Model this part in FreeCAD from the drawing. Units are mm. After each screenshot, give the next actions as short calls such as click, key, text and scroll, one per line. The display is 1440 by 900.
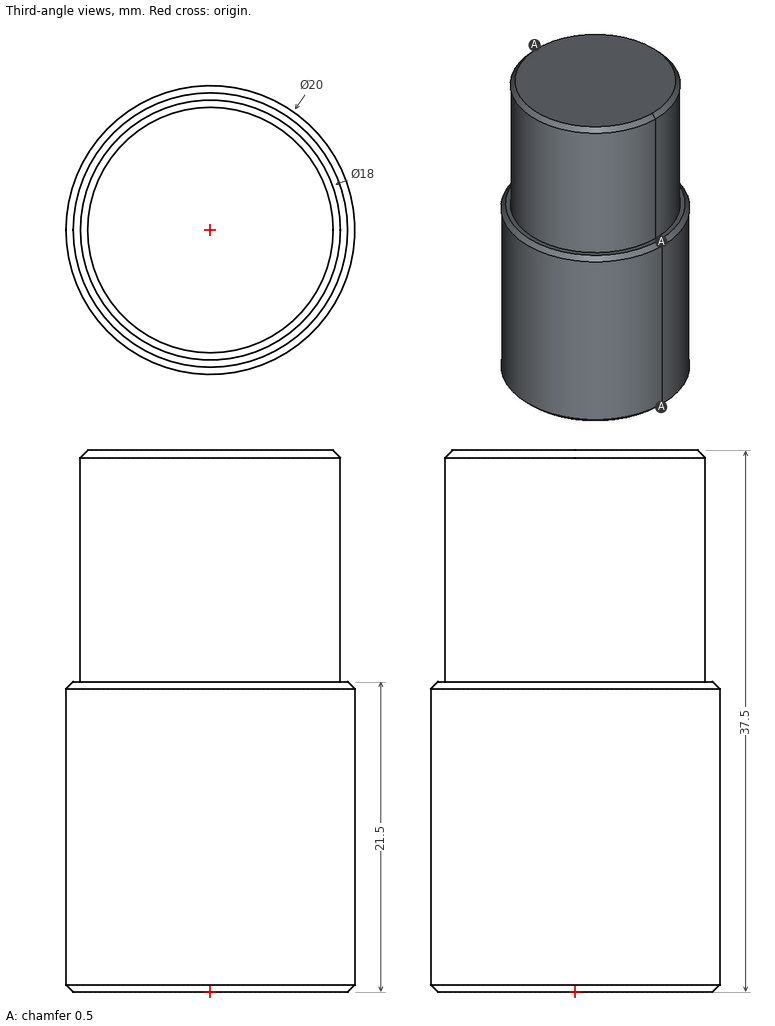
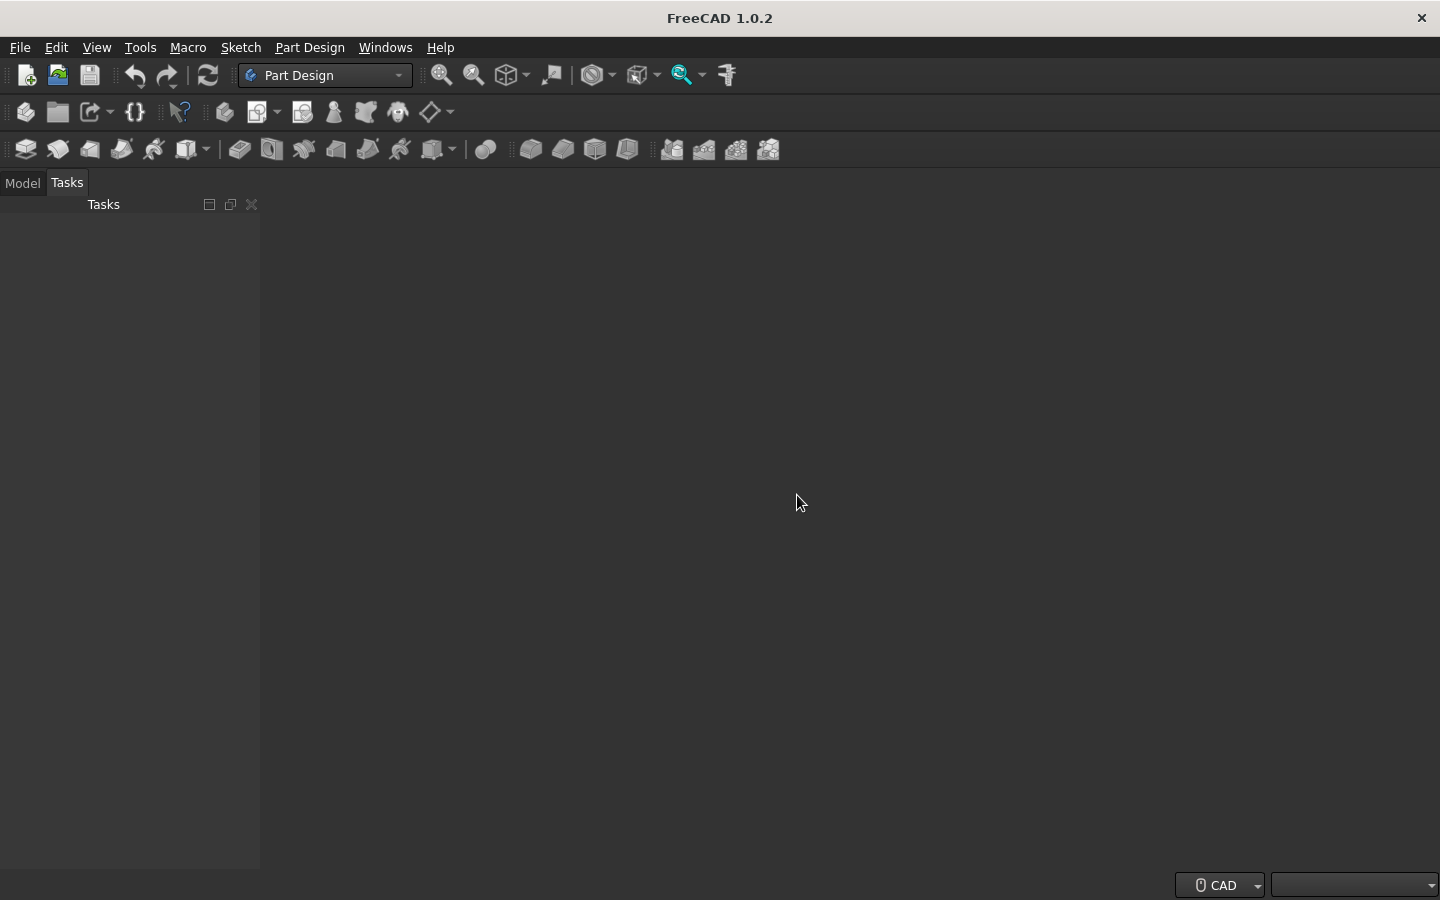
click(26, 76)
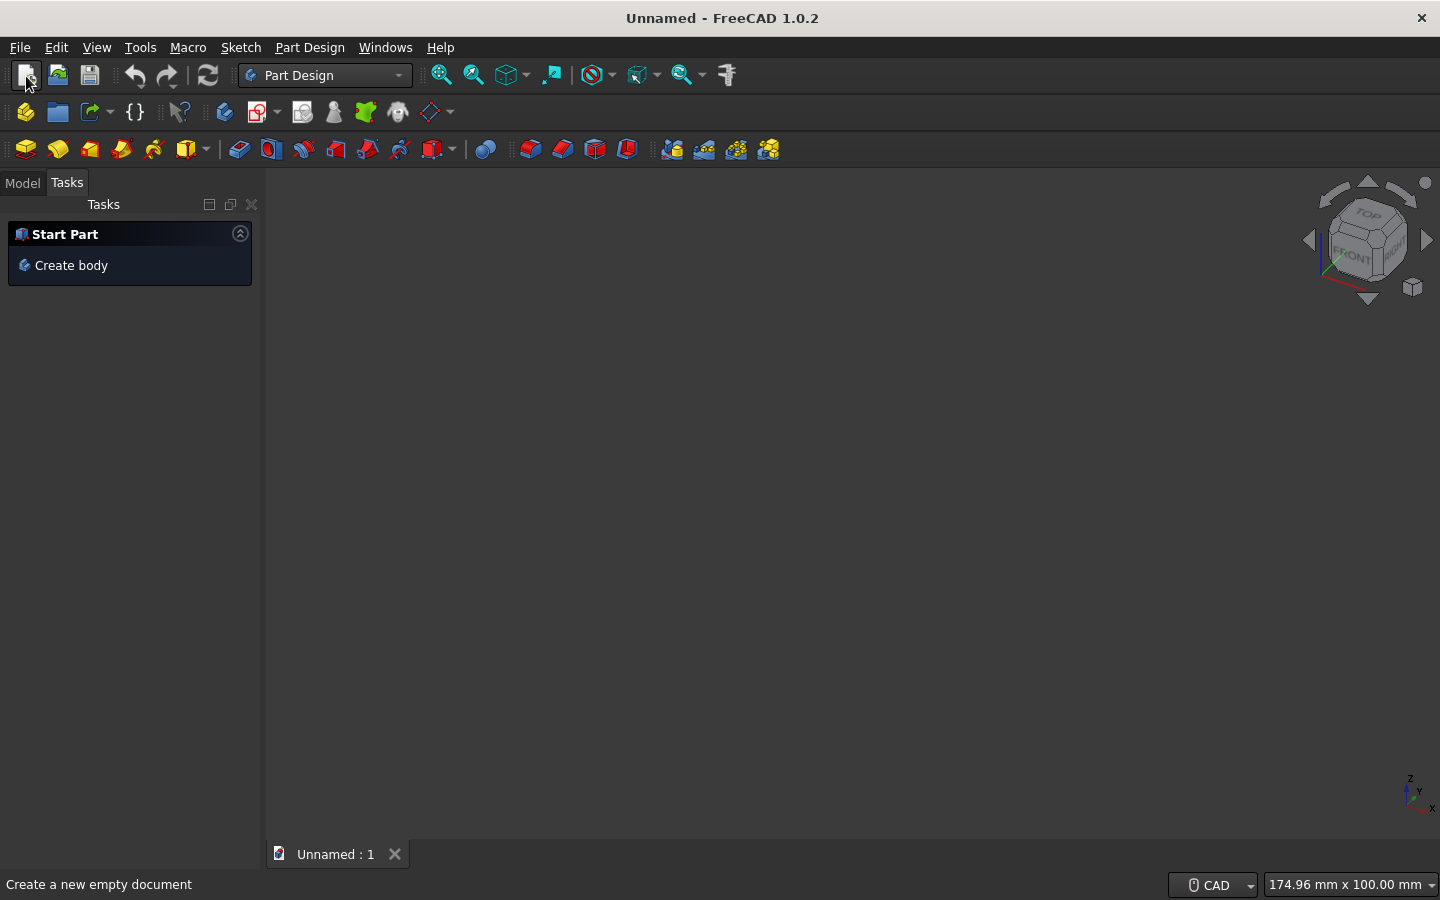
click(258, 112)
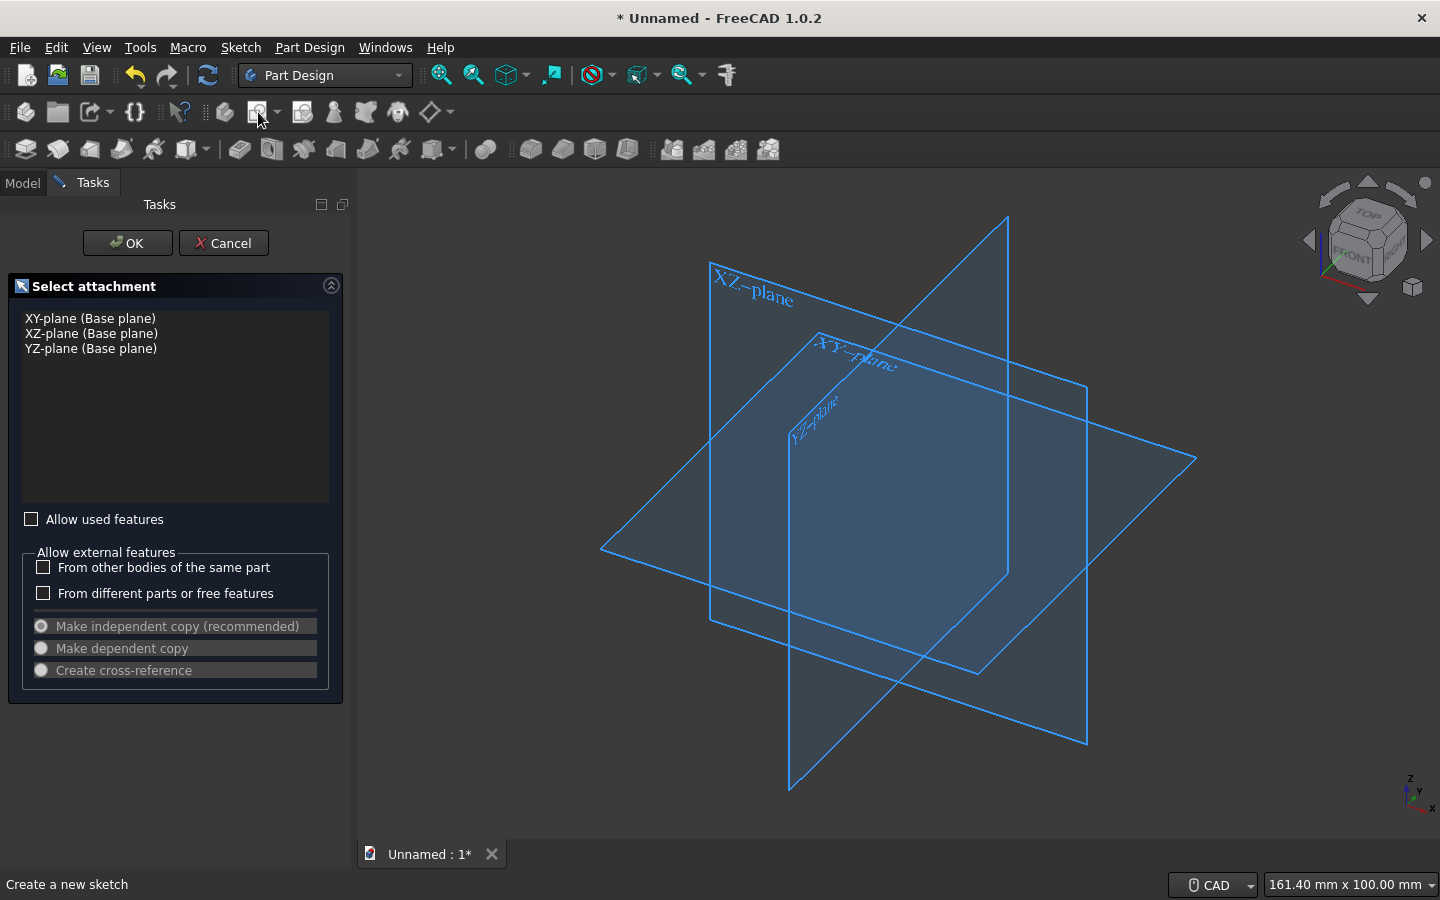
click(82, 318)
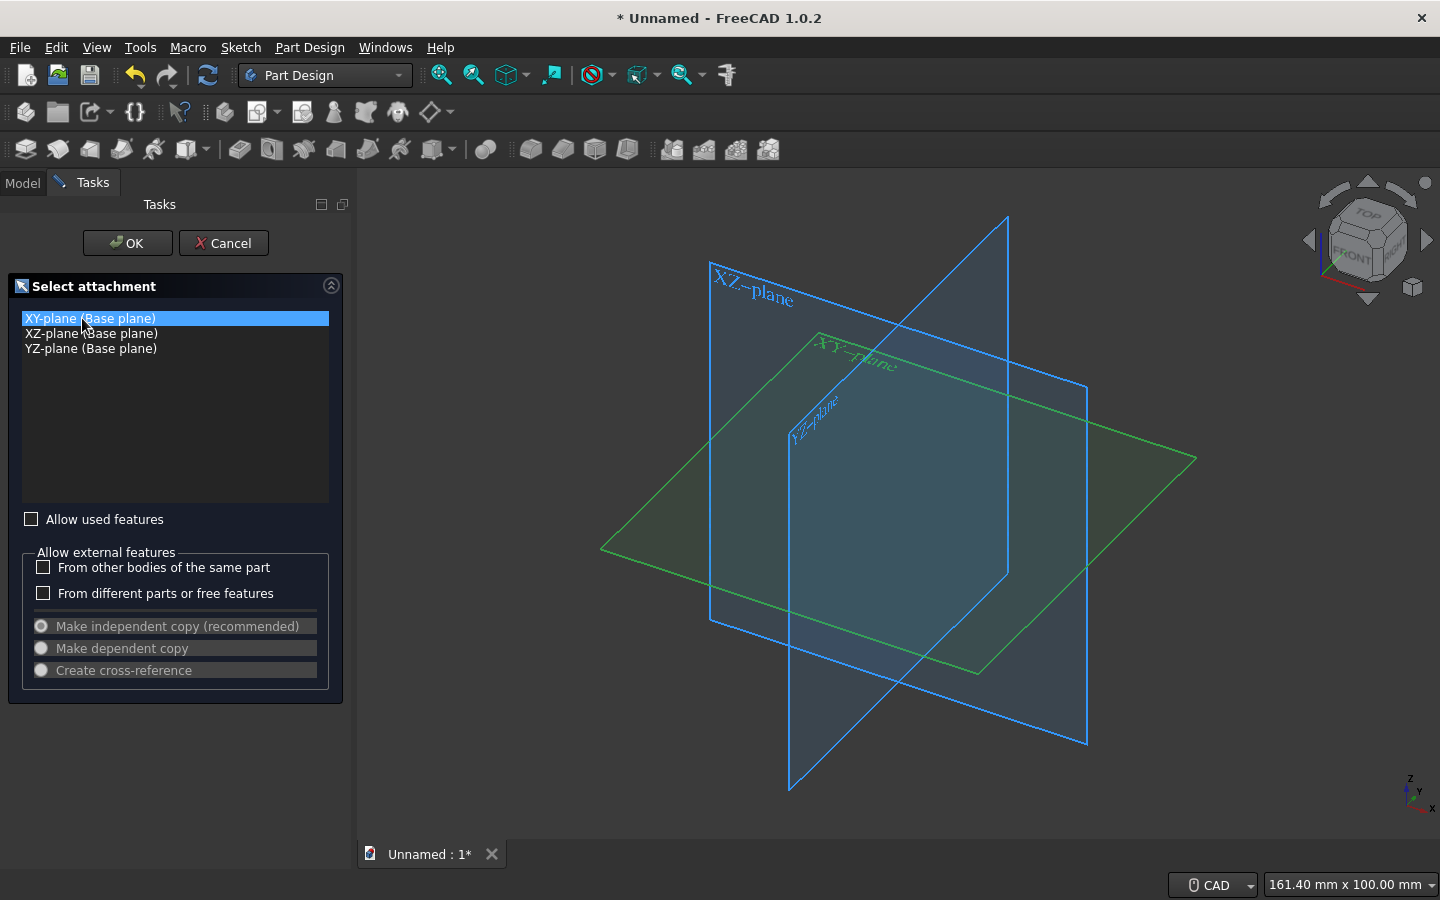
click(128, 243)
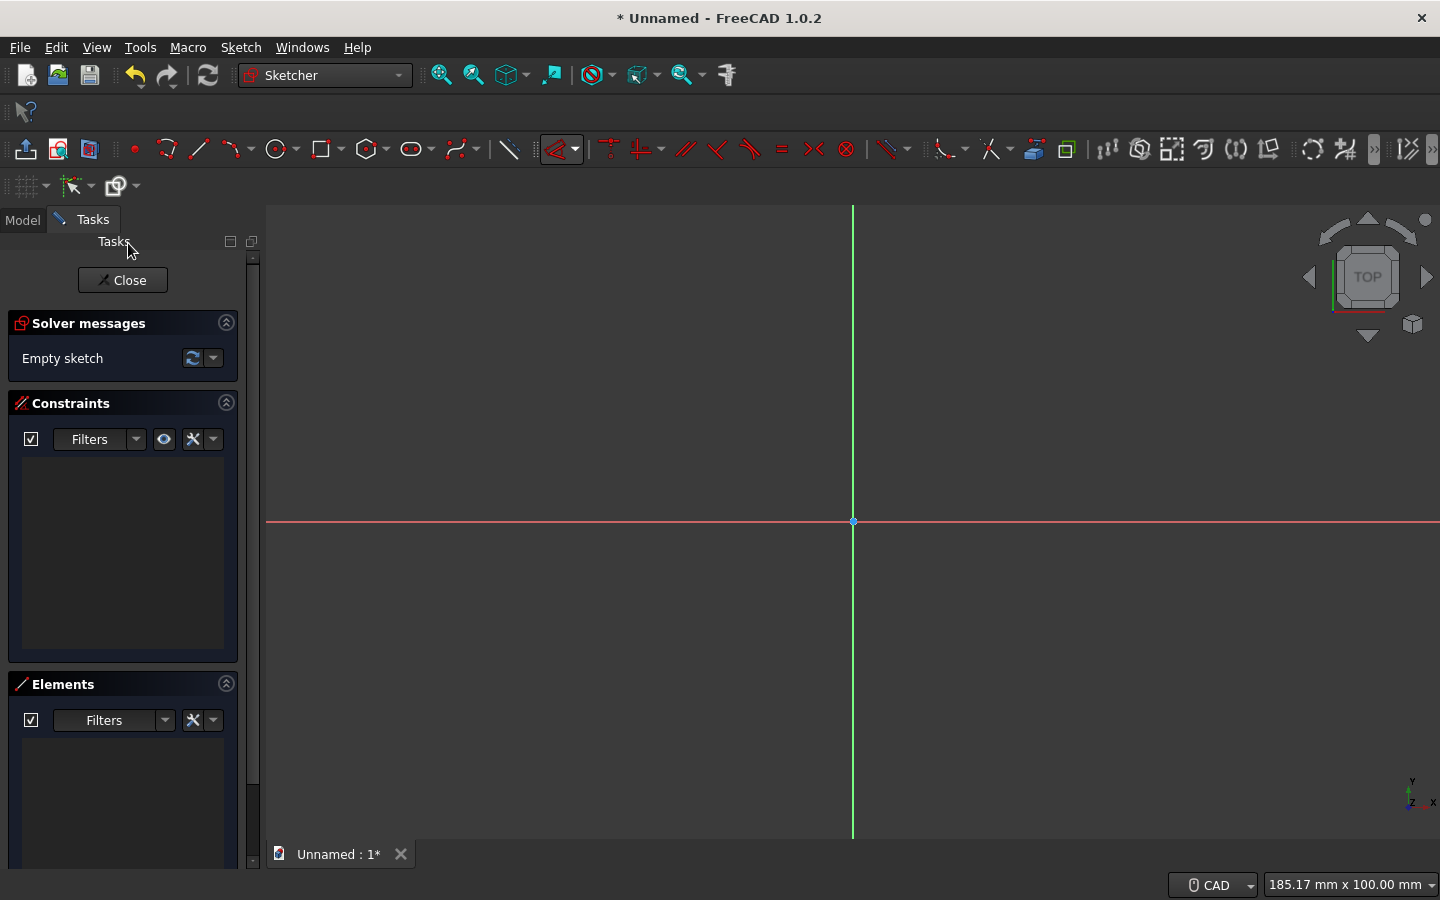
scroll(883, 522, up, 6)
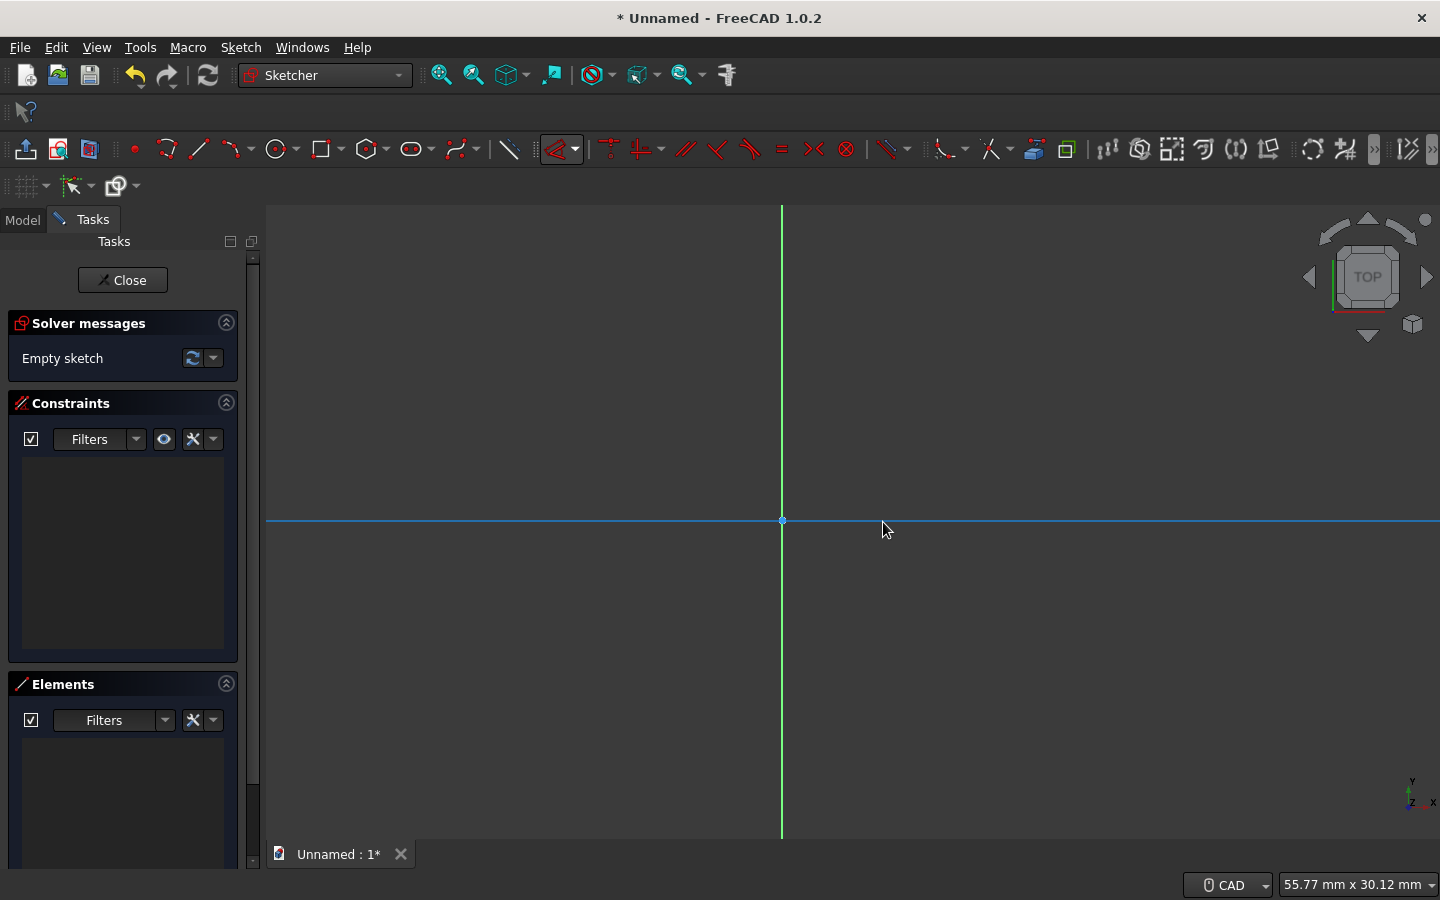
click(276, 150)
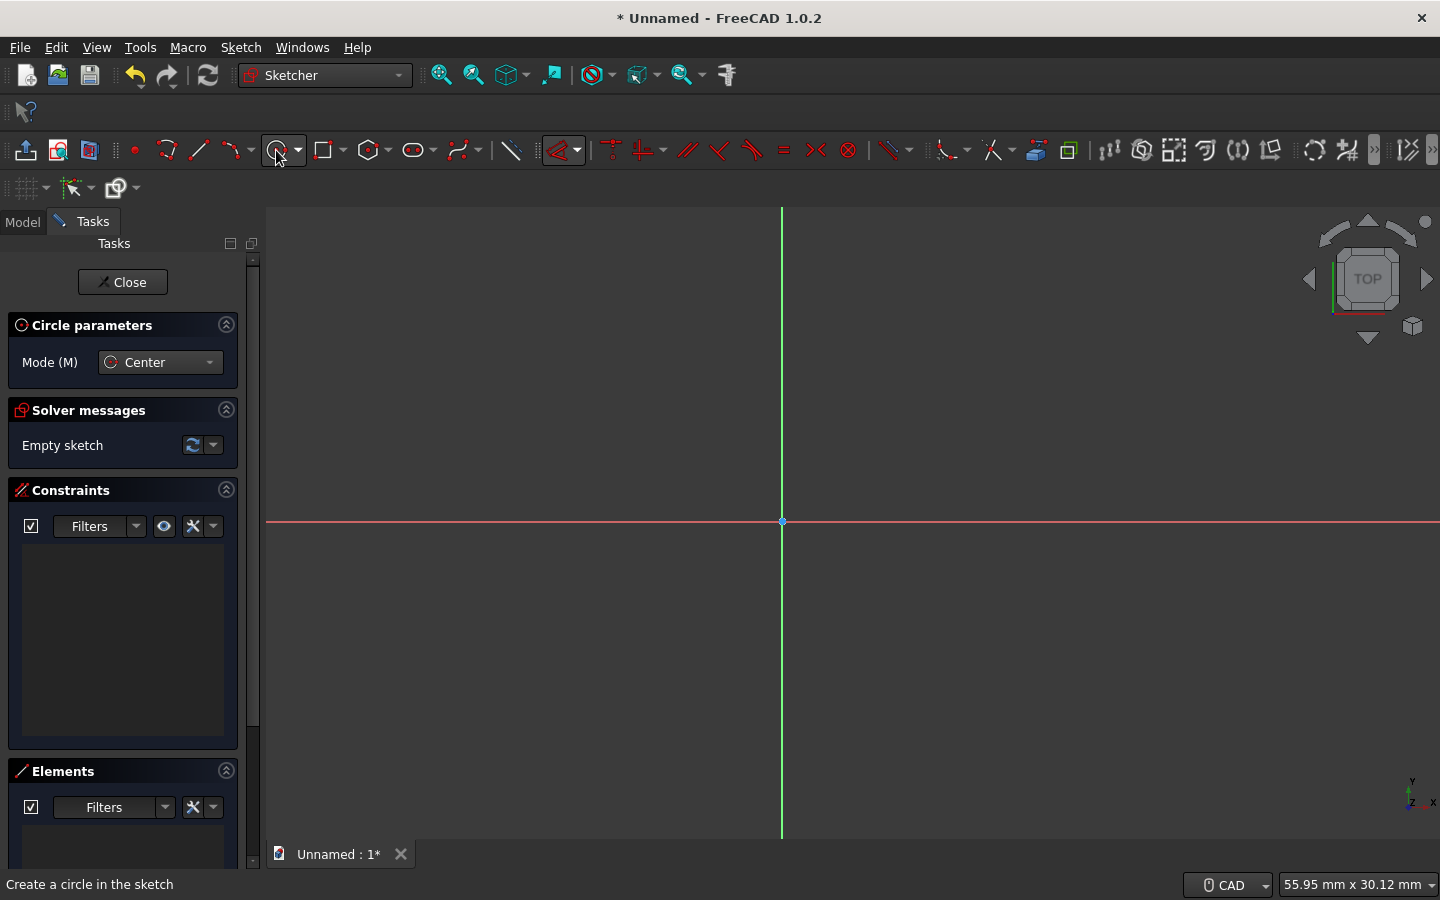
click(782, 522)
move(916, 388)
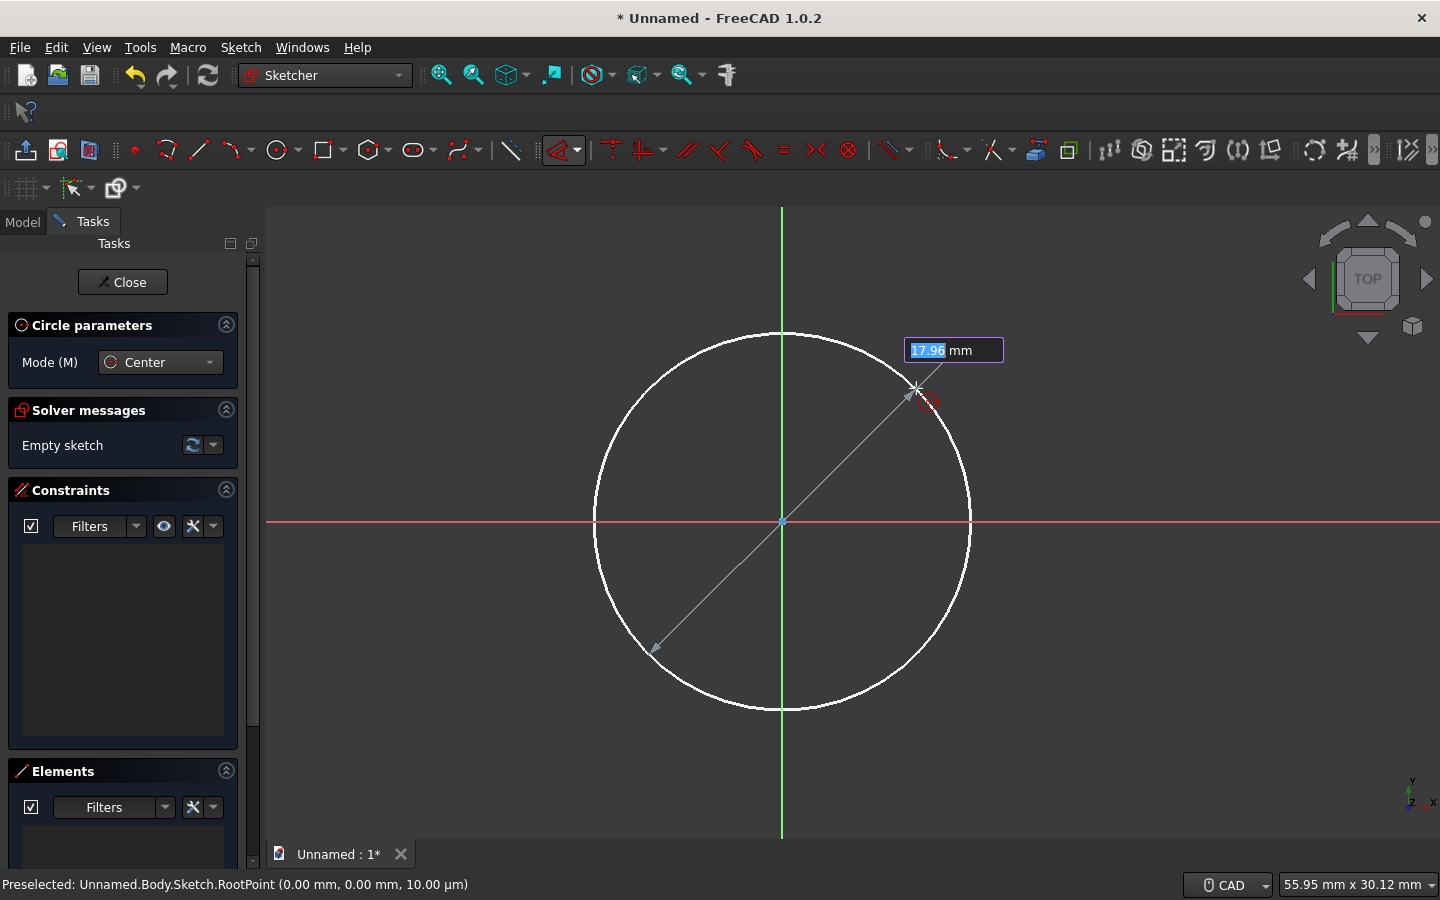
text(18)
key(Return)
key(Escape)